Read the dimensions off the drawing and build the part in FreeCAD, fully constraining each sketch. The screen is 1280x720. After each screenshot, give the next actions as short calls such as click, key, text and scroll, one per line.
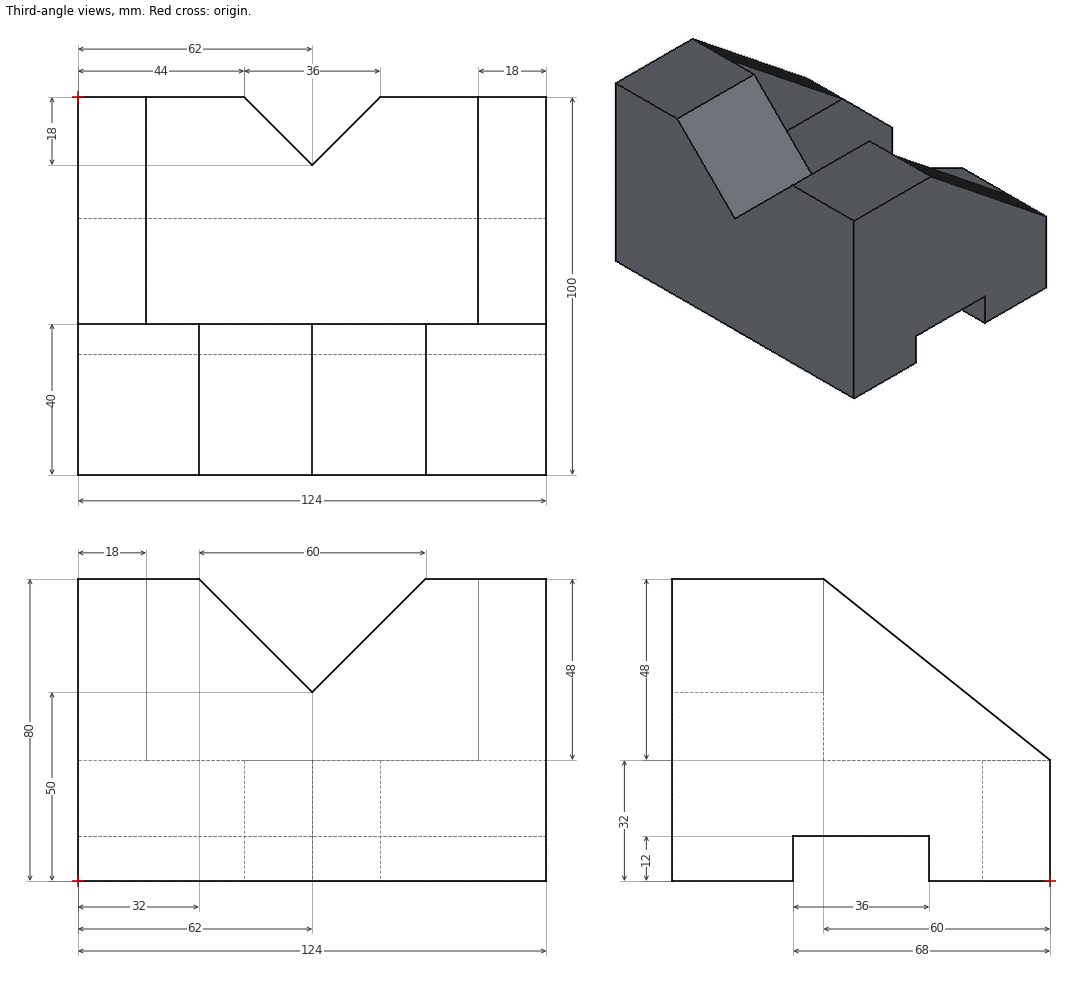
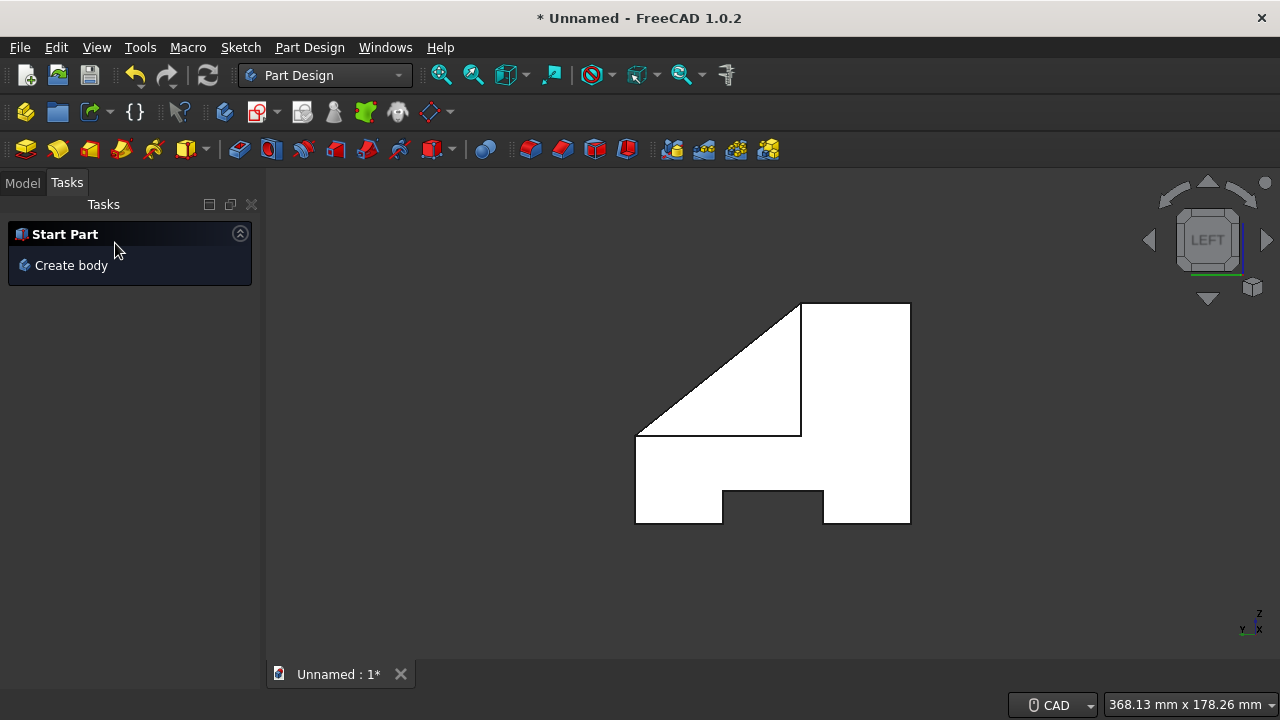
click(852, 444)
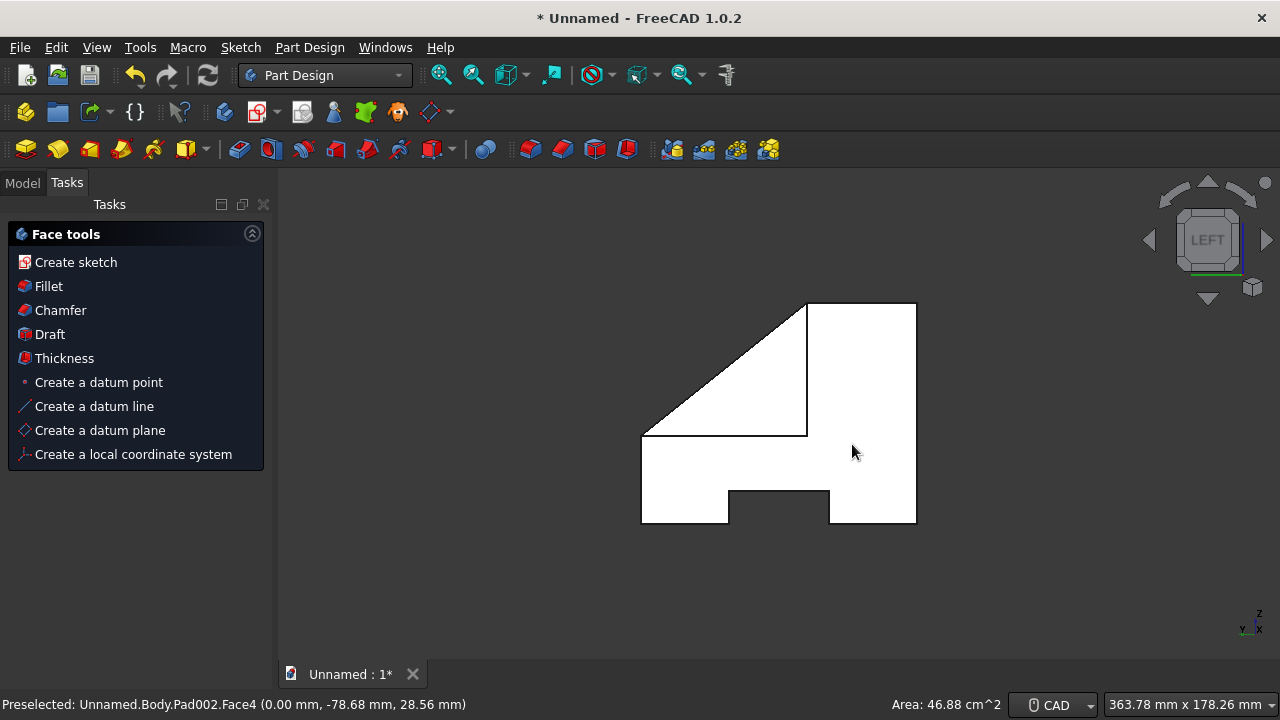
click(258, 112)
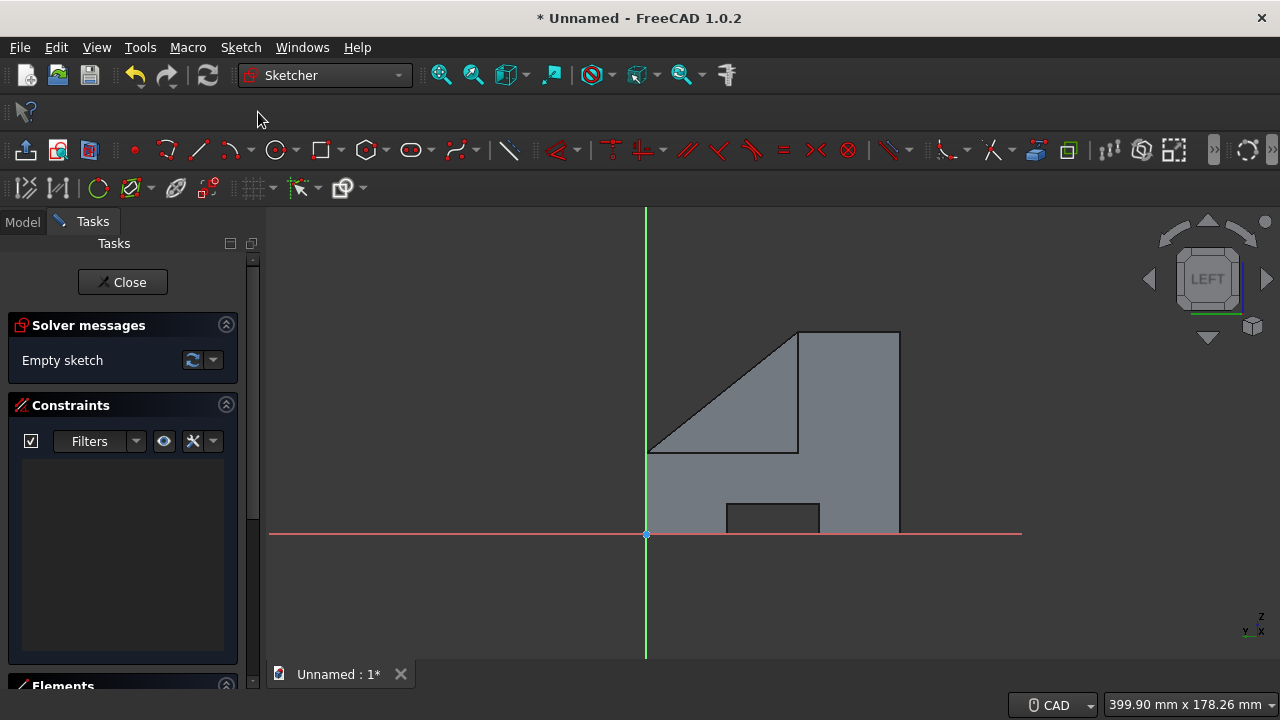
scroll(758, 433, up, 2)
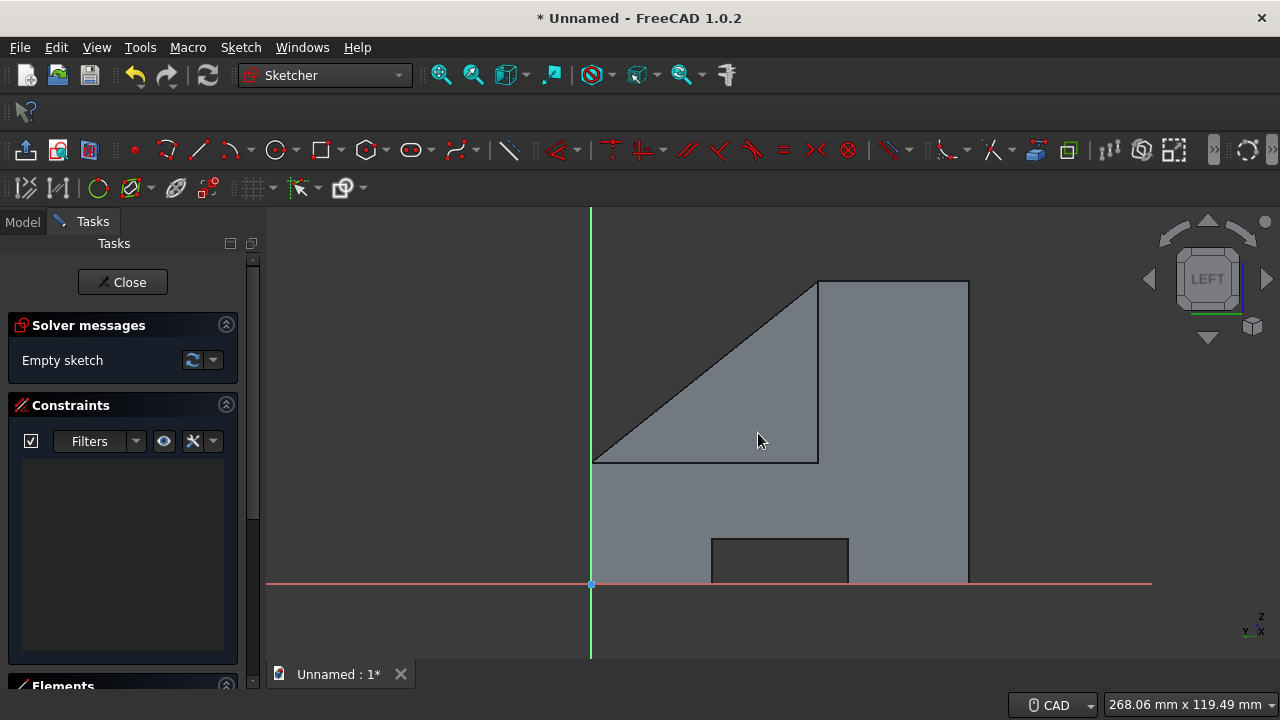
key(g)
key(m)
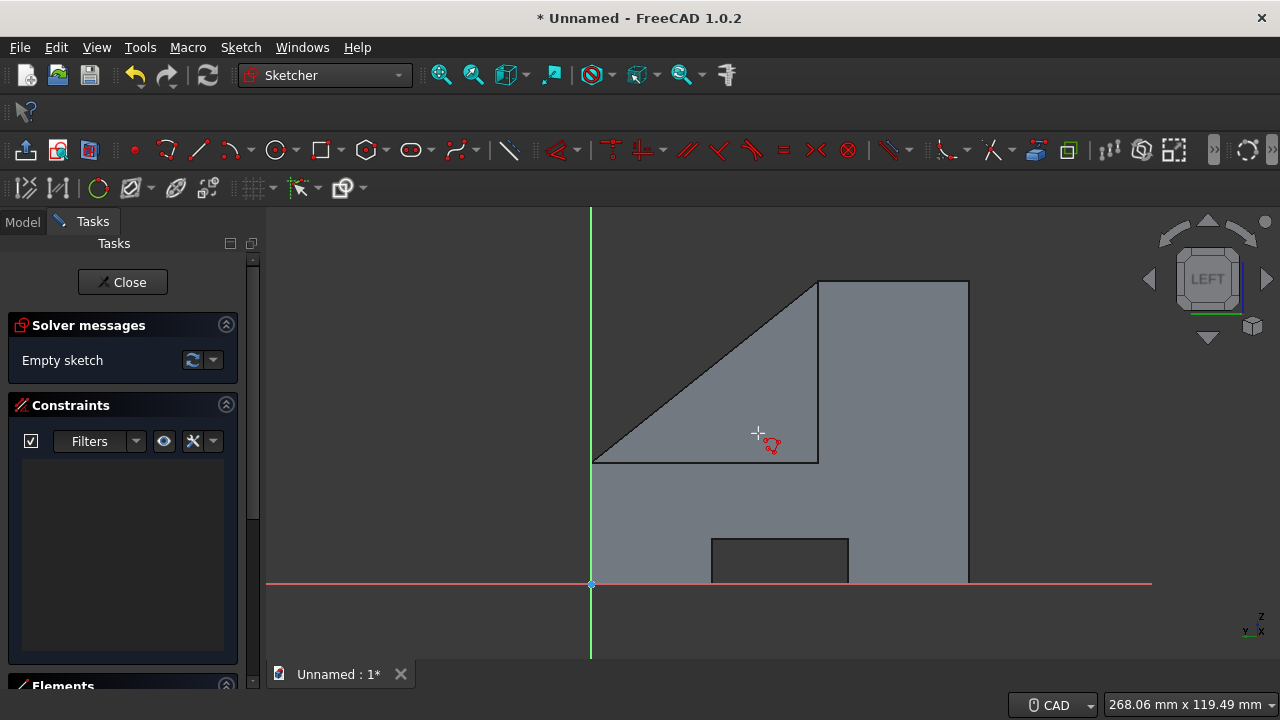
click(591, 463)
click(818, 463)
click(818, 281)
click(591, 464)
key(Escape)
key(Escape)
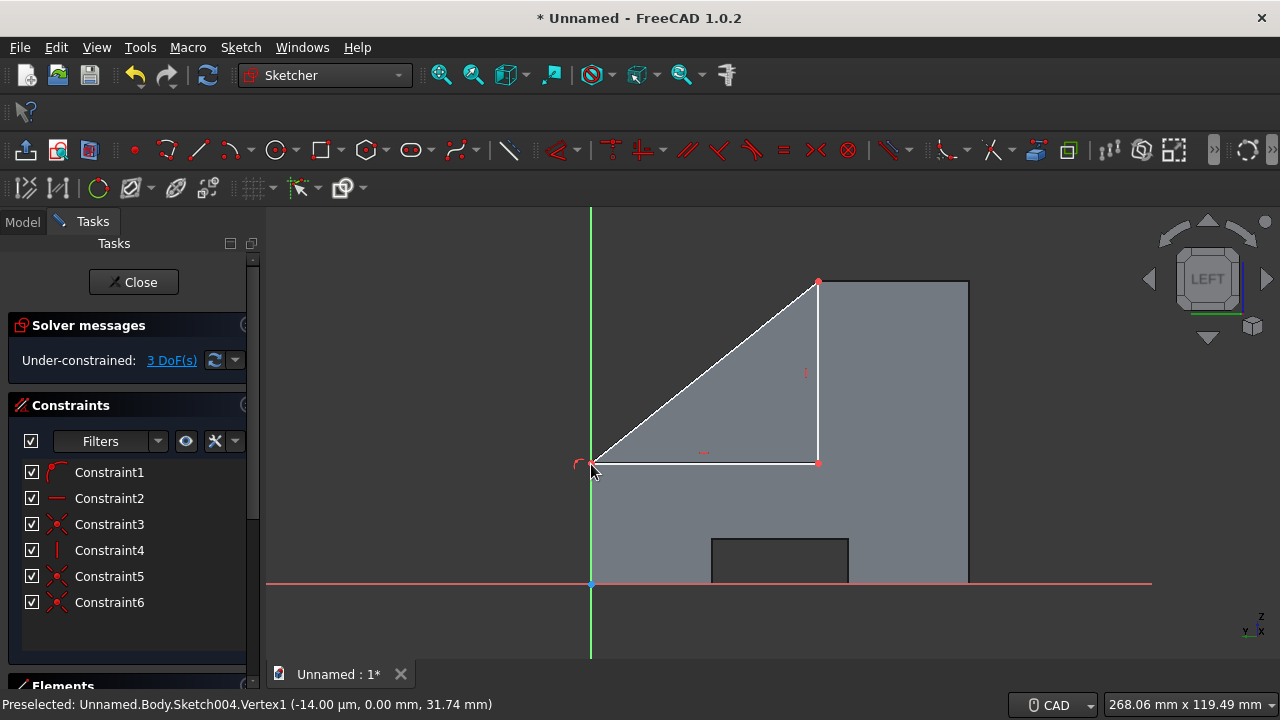
click(556, 150)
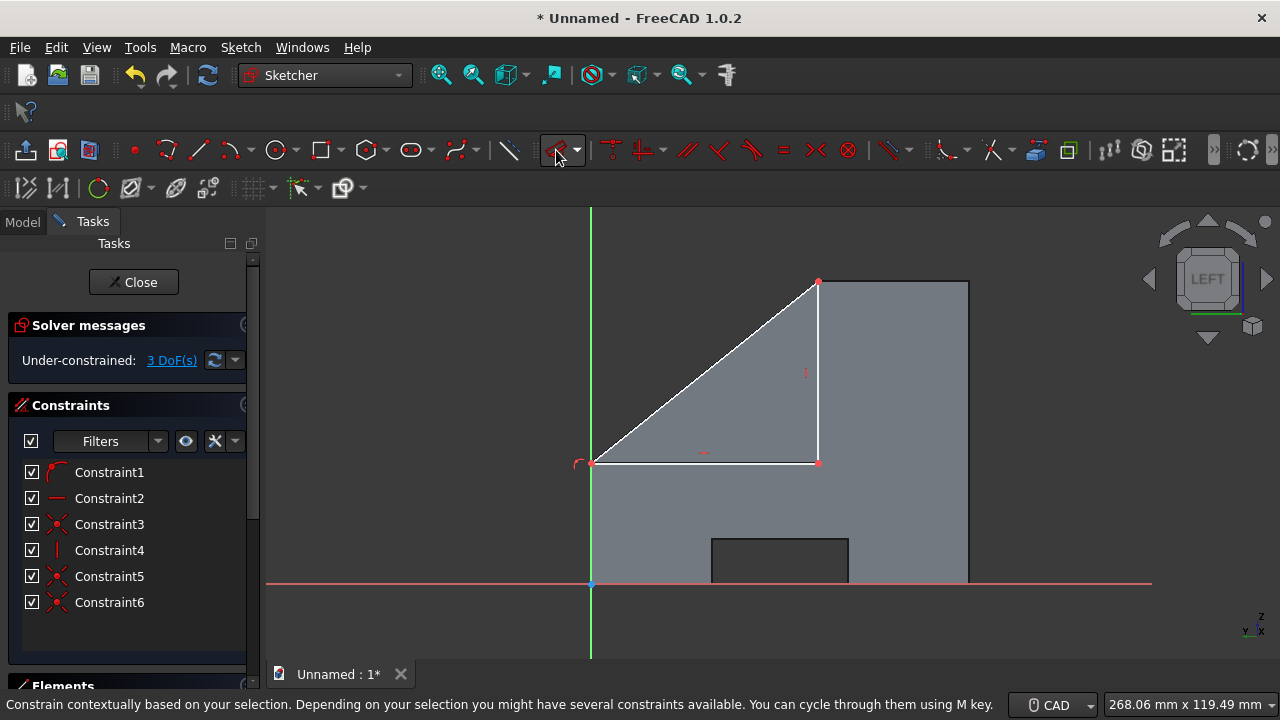
click(659, 464)
click(705, 498)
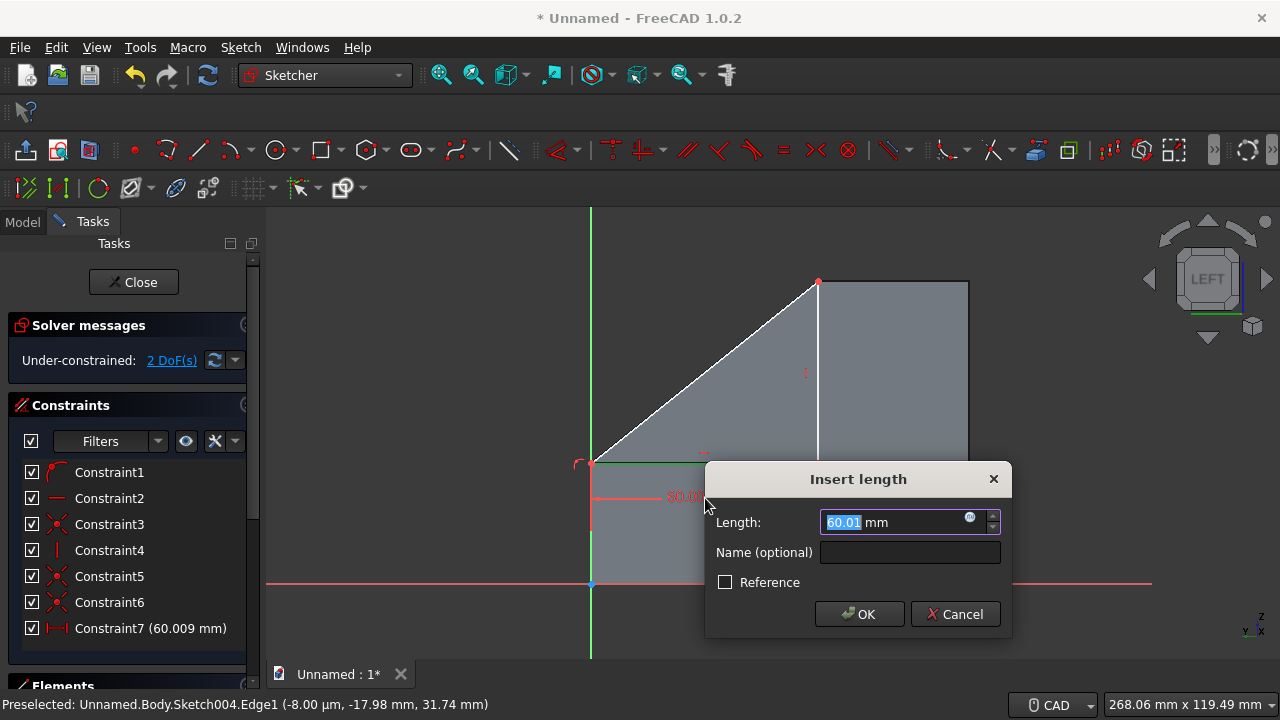
text(60)
key(Return)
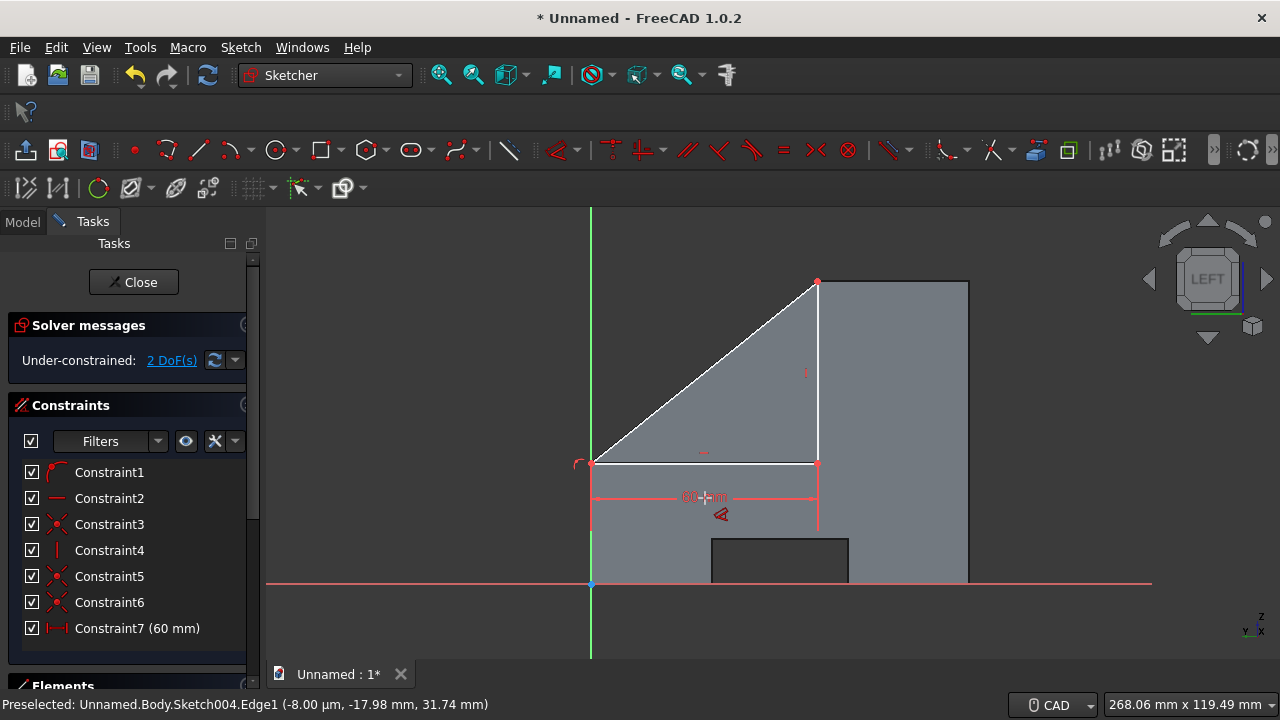
click(818, 409)
click(852, 373)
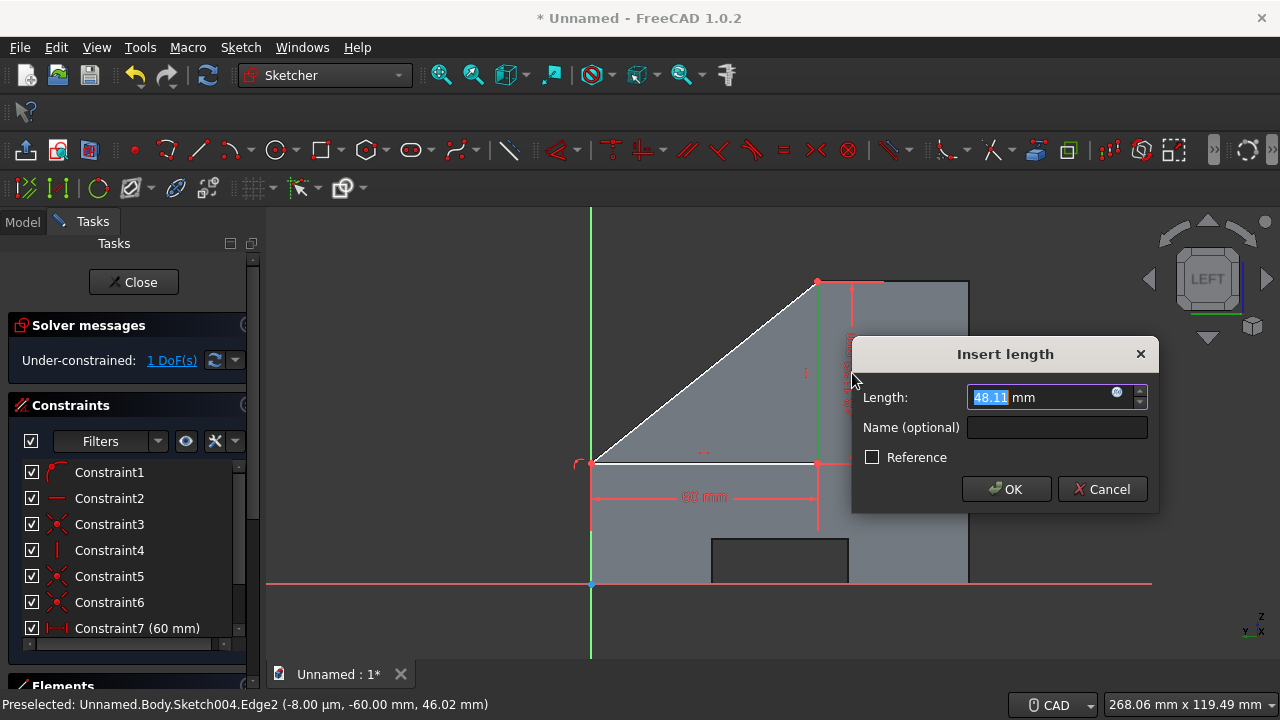
text(48)
key(Return)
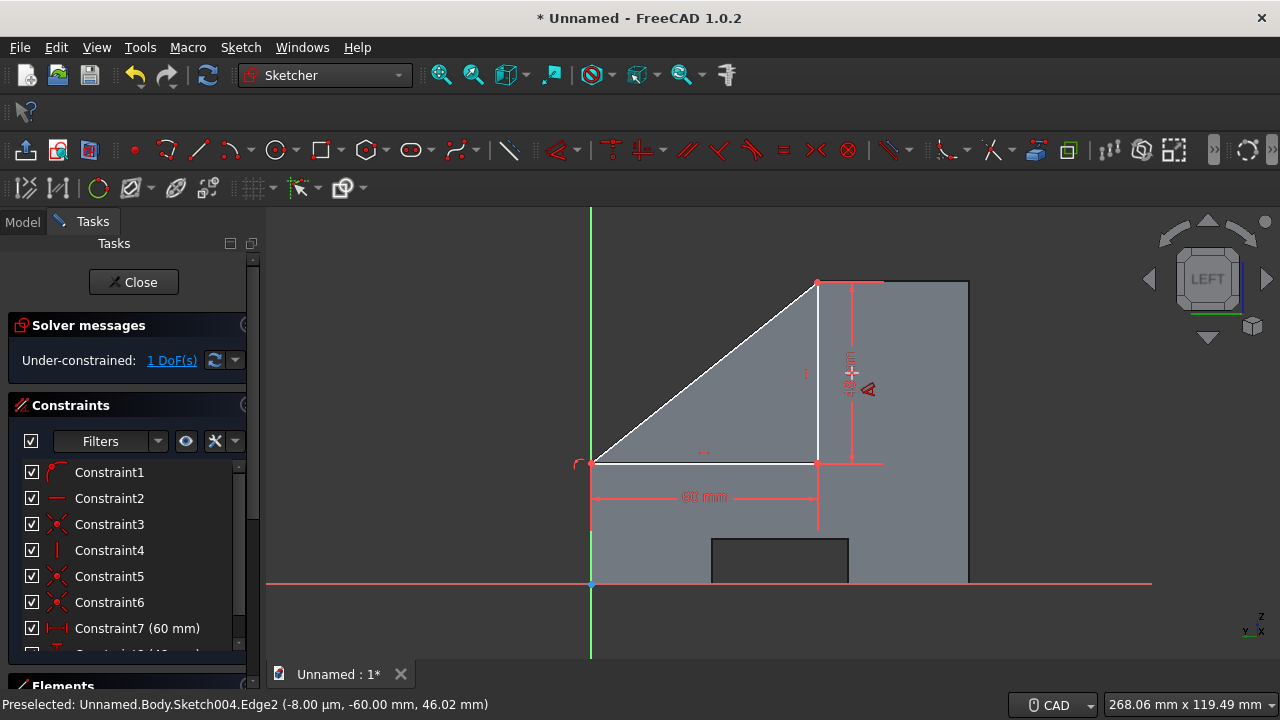
click(591, 464)
click(557, 524)